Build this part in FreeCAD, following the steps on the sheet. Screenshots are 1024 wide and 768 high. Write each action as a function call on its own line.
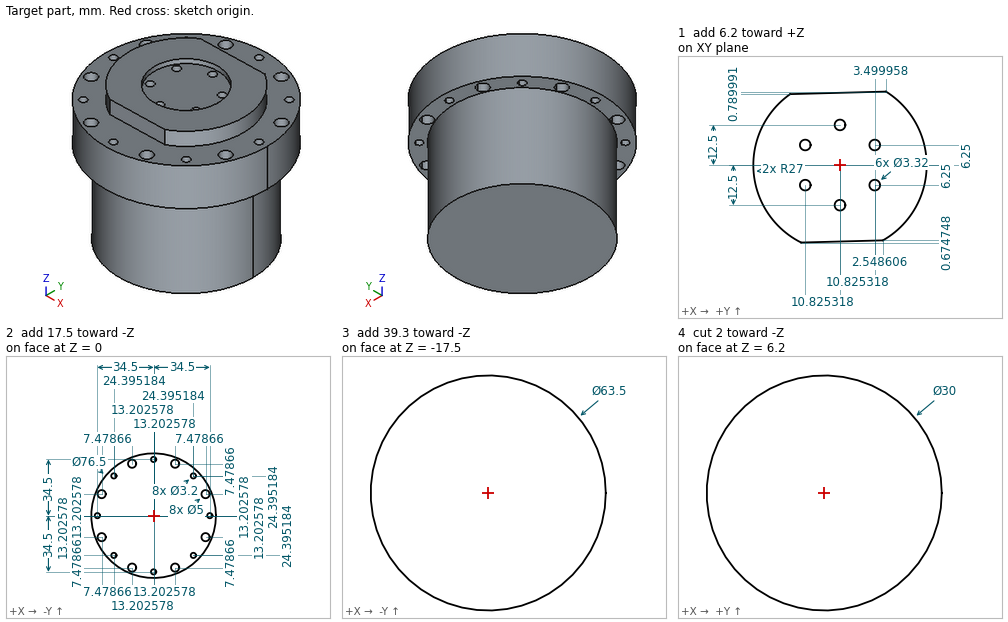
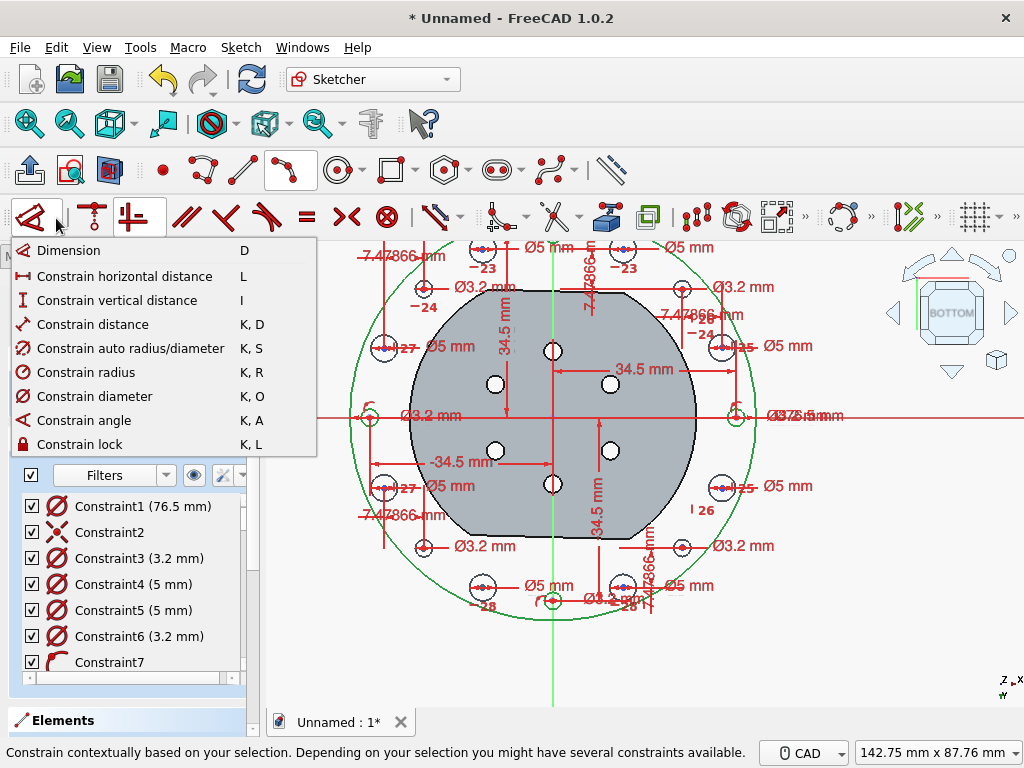
click(164, 300)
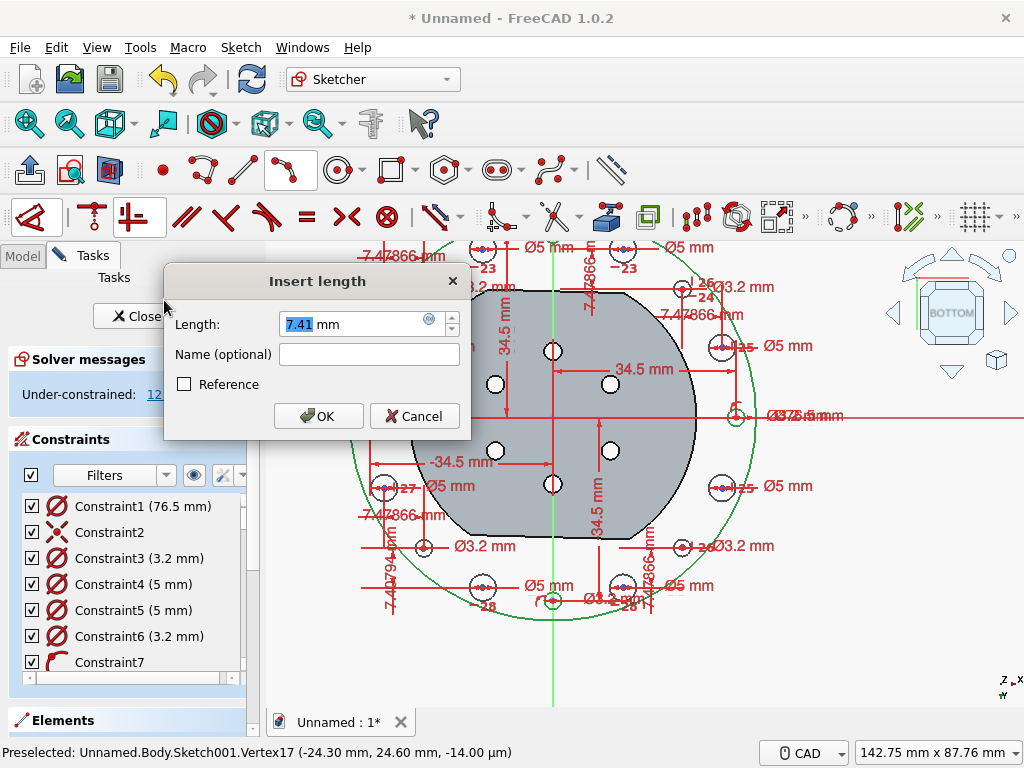
text(7.47866)
key(Return)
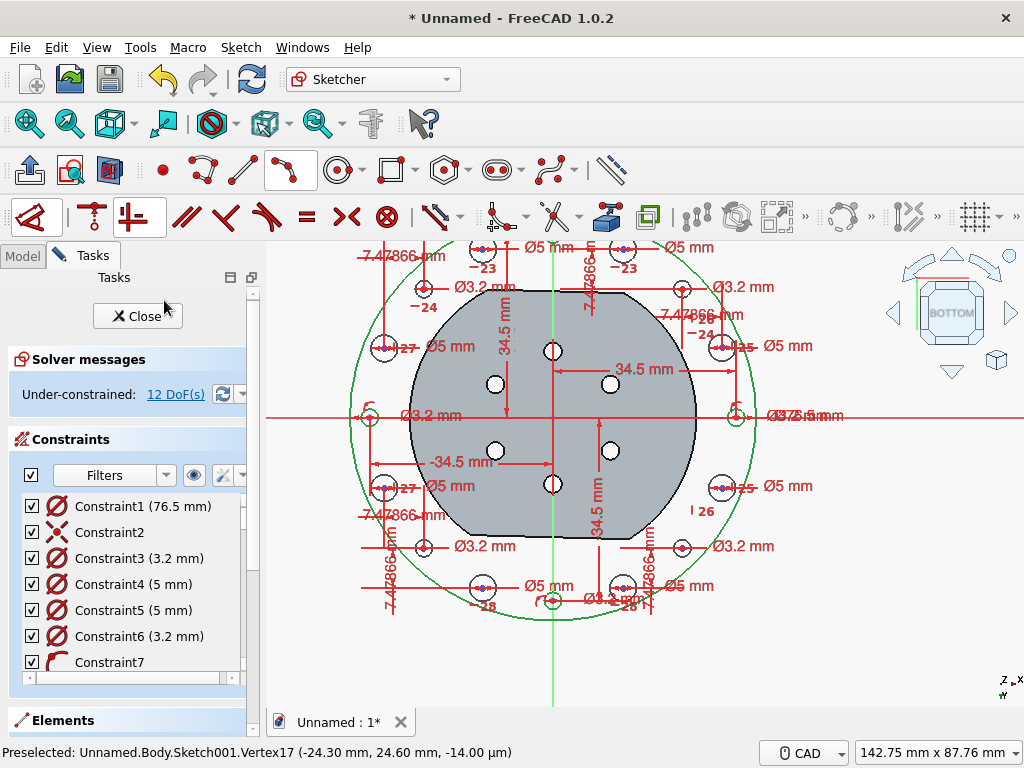
click(682, 289)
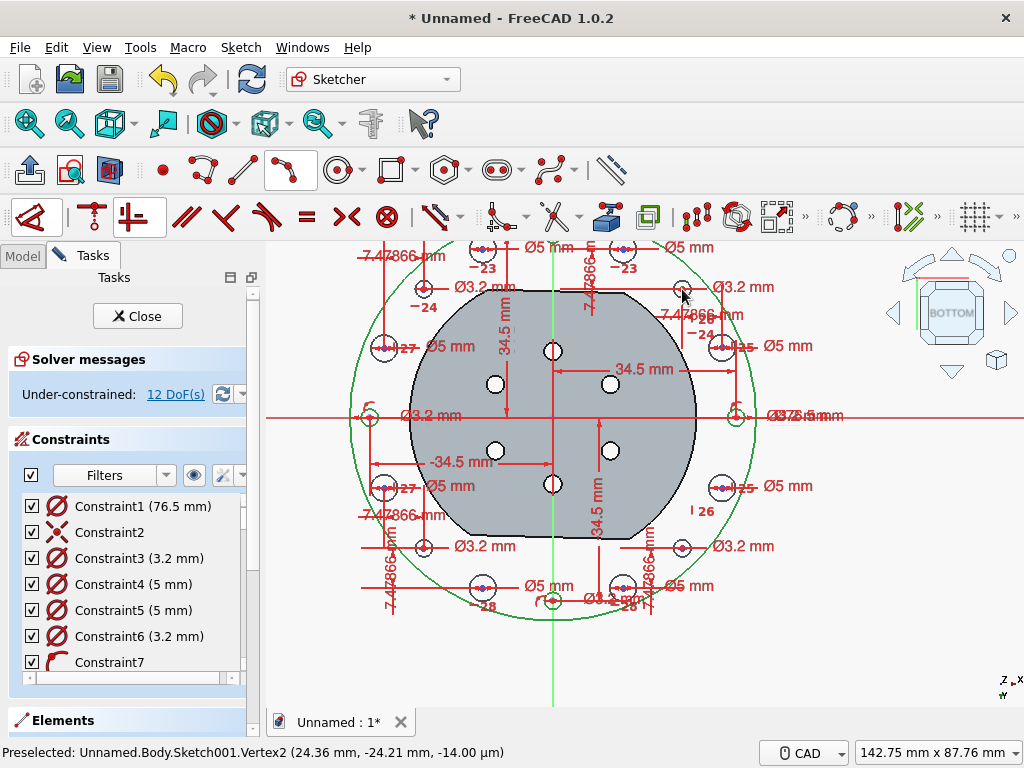
key(l)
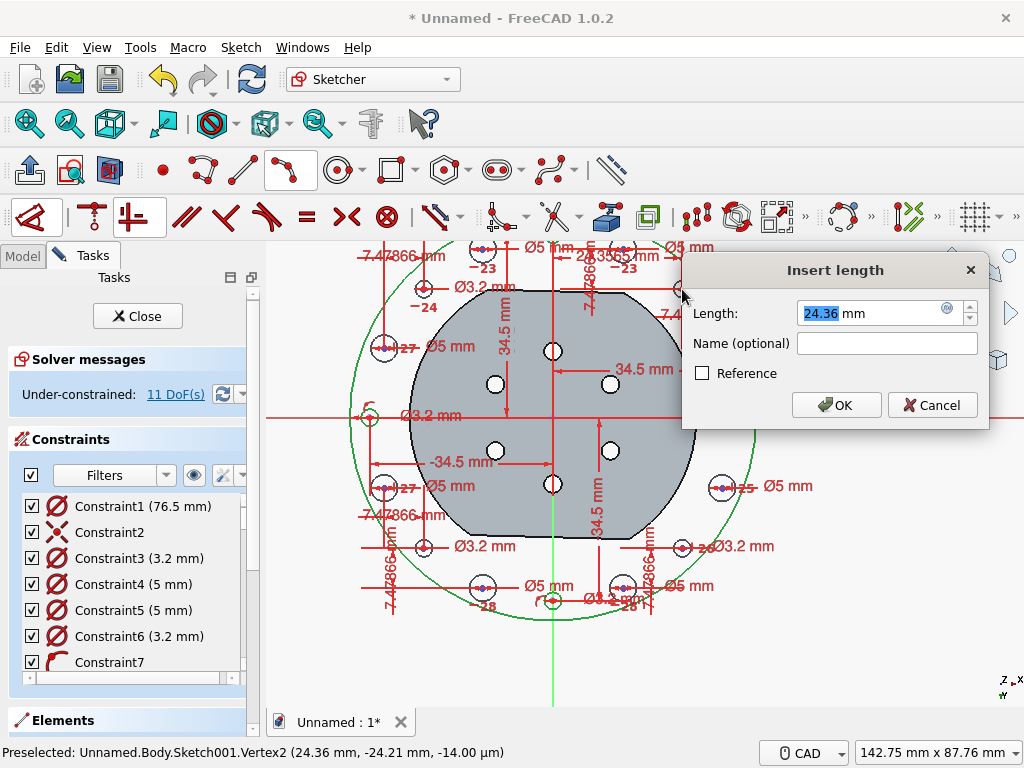
text(24.395184)
key(Return)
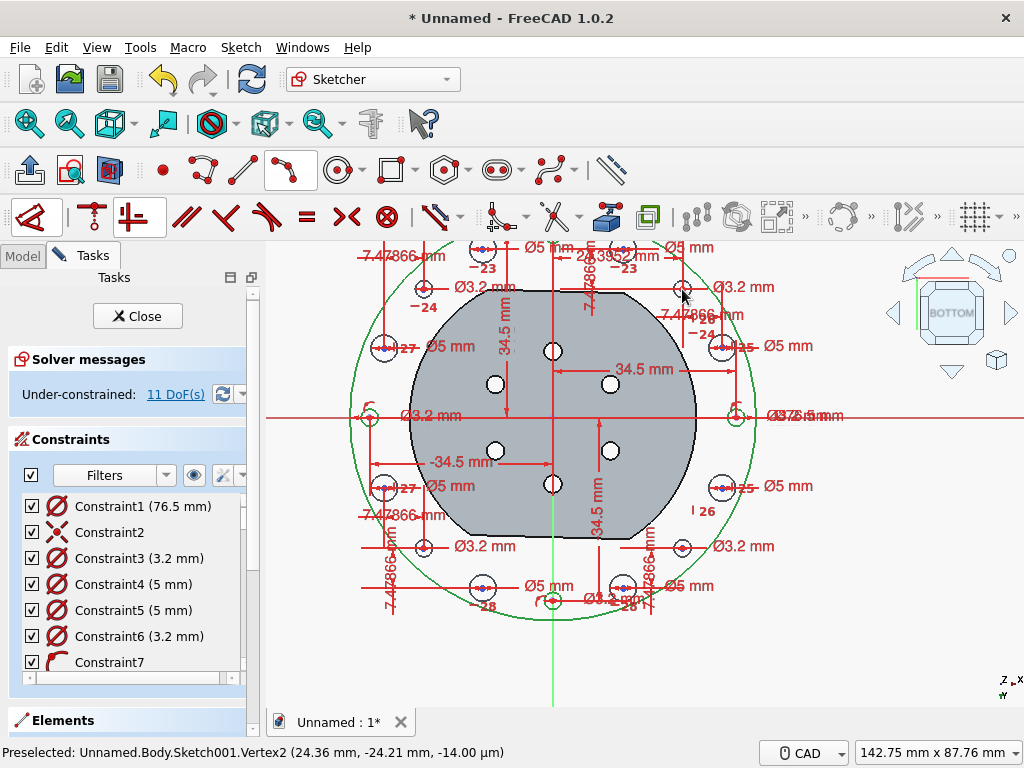
click(683, 289)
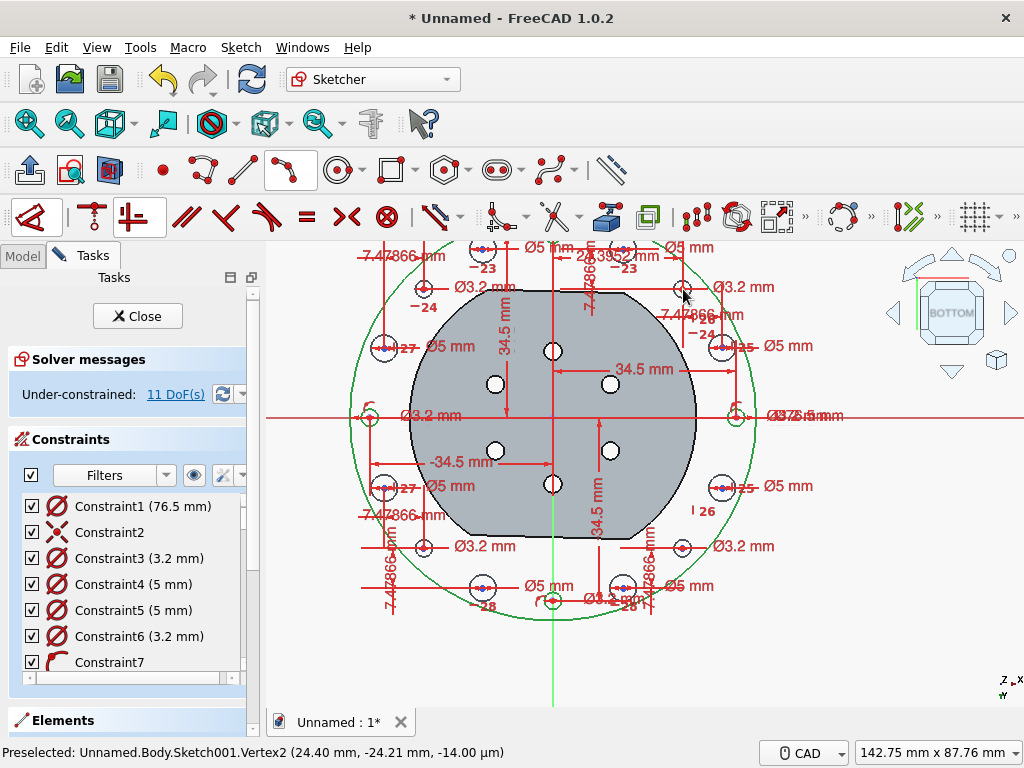
click(56, 218)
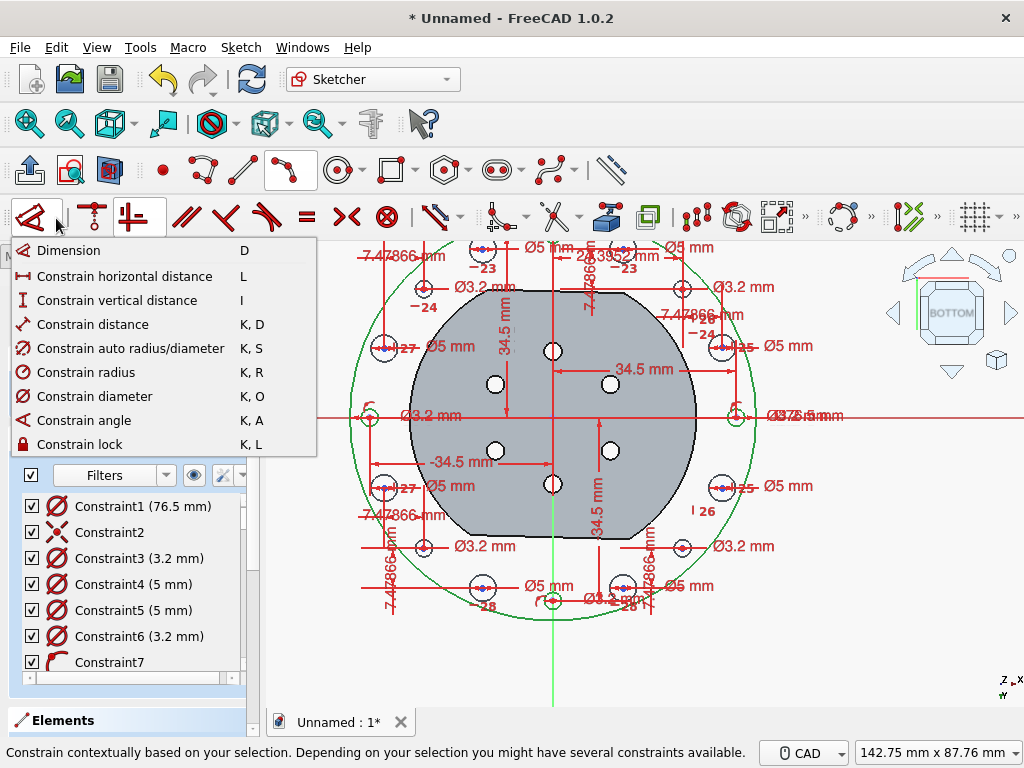
click(164, 300)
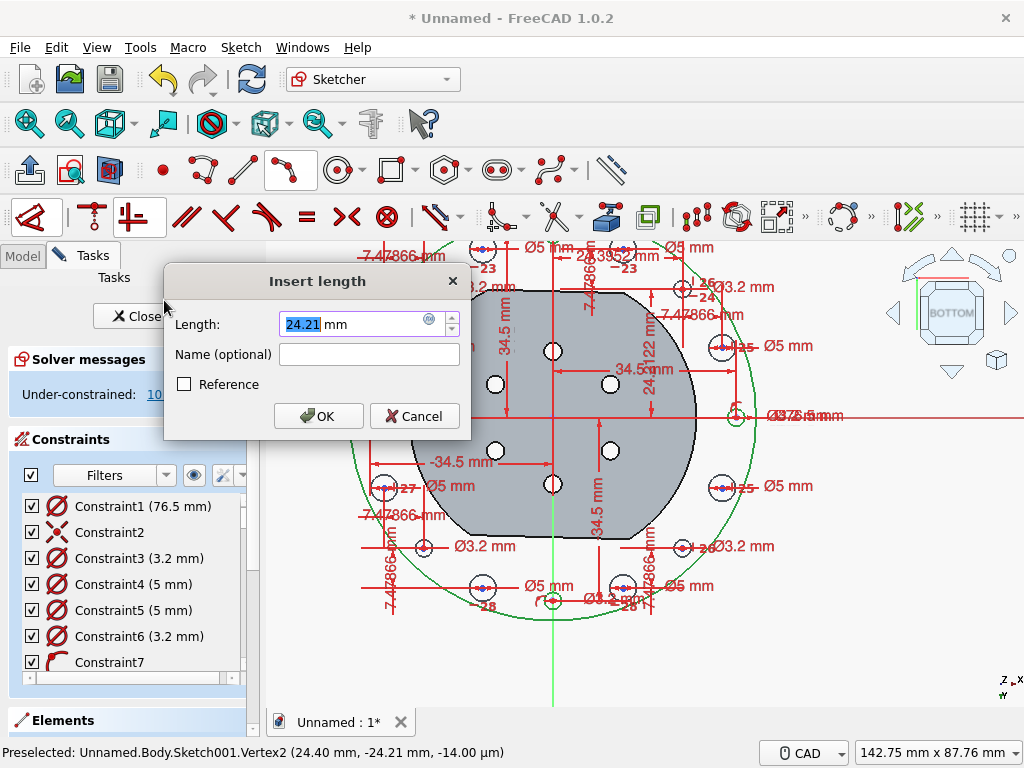
text(24.395184)
key(Return)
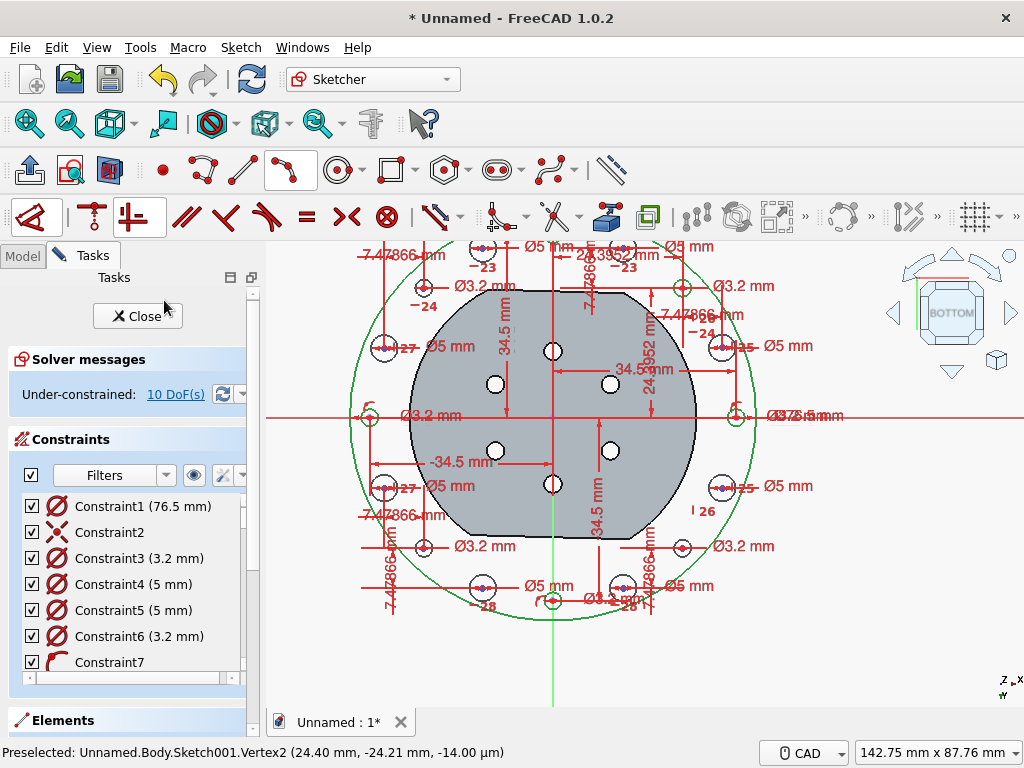
scroll(624, 588, down, 2)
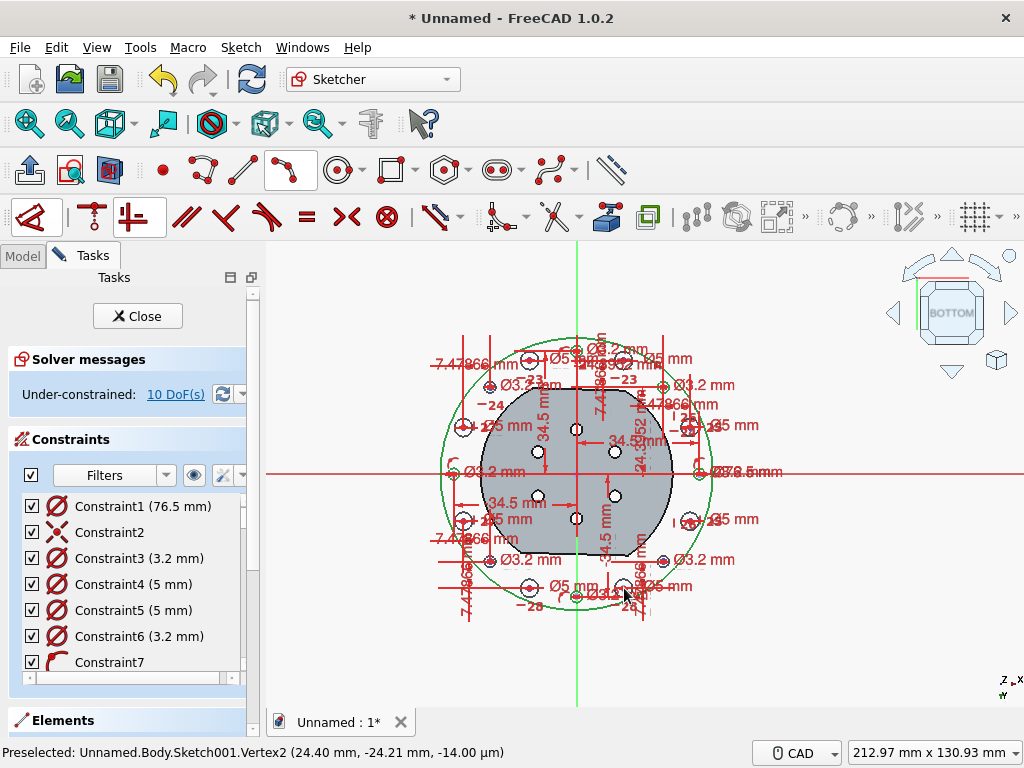
click(624, 361)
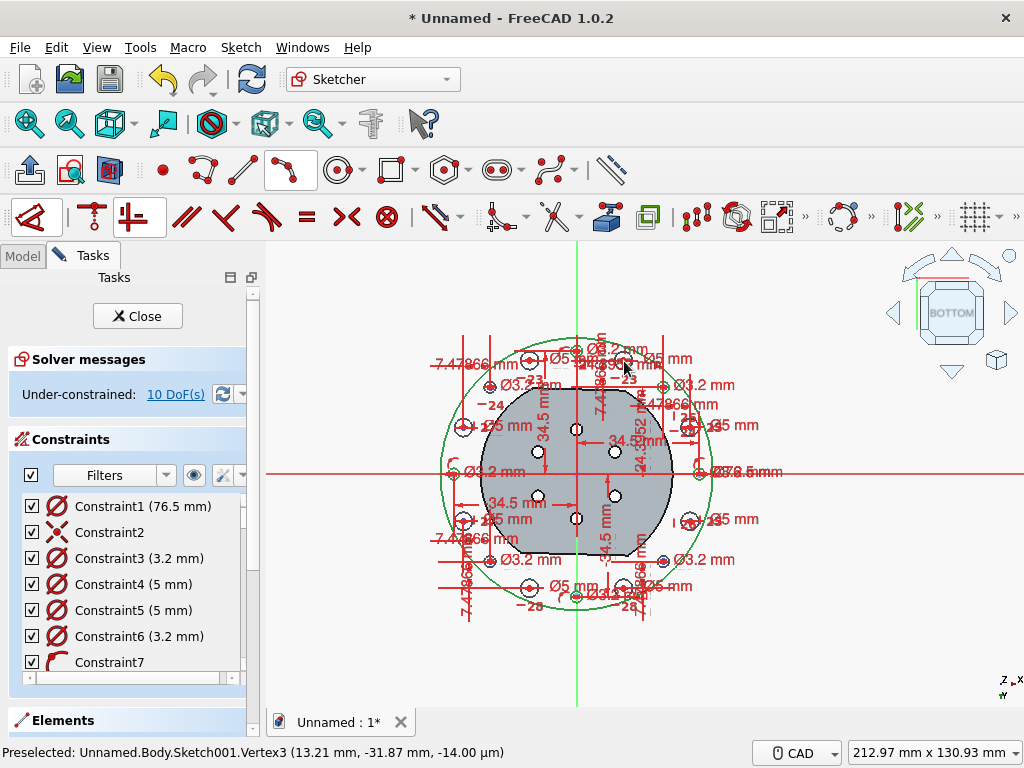
key(l)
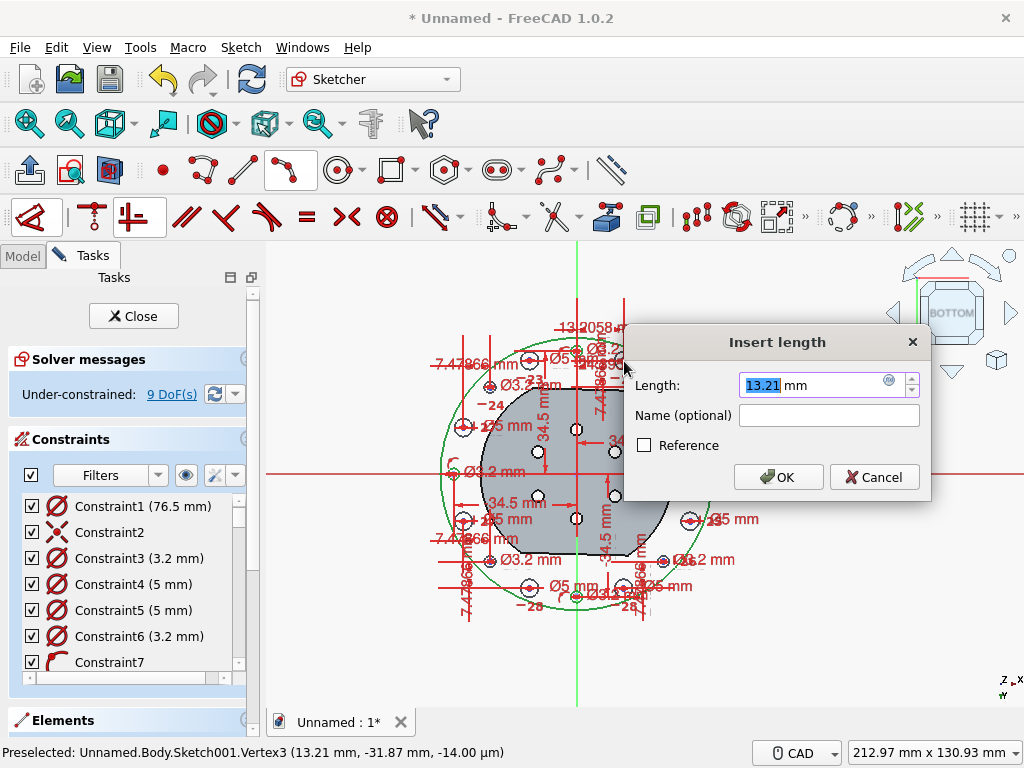
text(13.202578)
key(Return)